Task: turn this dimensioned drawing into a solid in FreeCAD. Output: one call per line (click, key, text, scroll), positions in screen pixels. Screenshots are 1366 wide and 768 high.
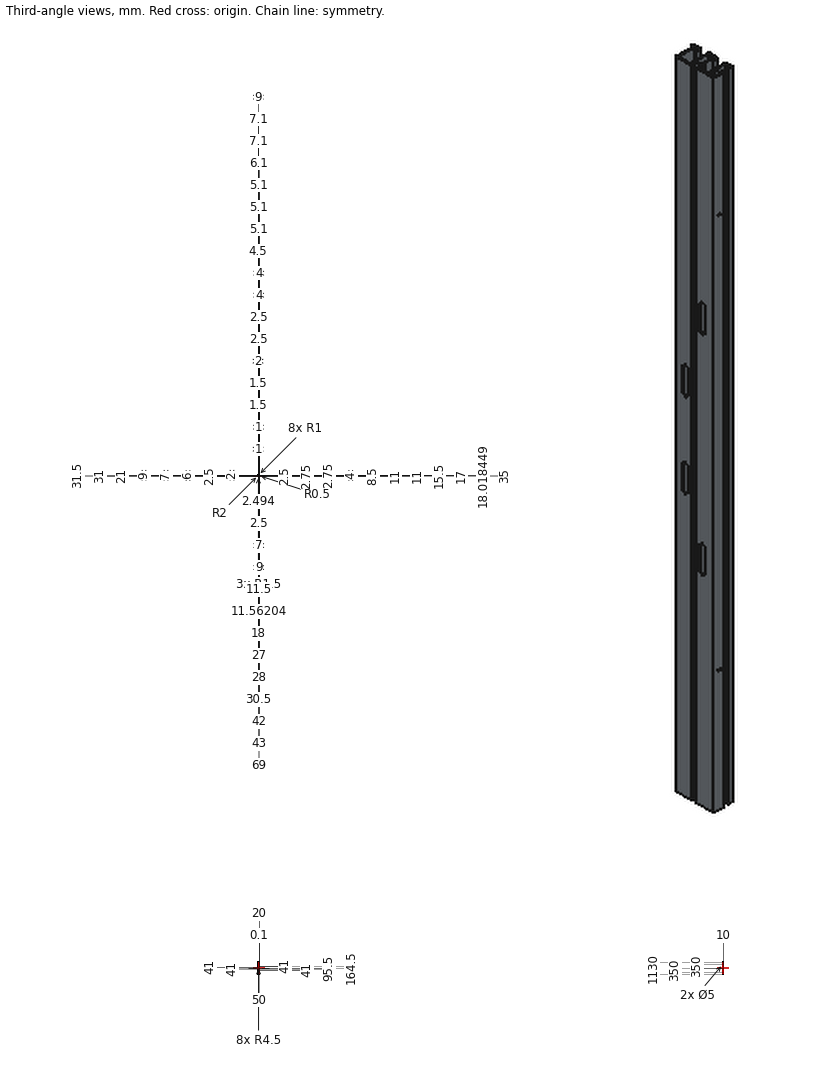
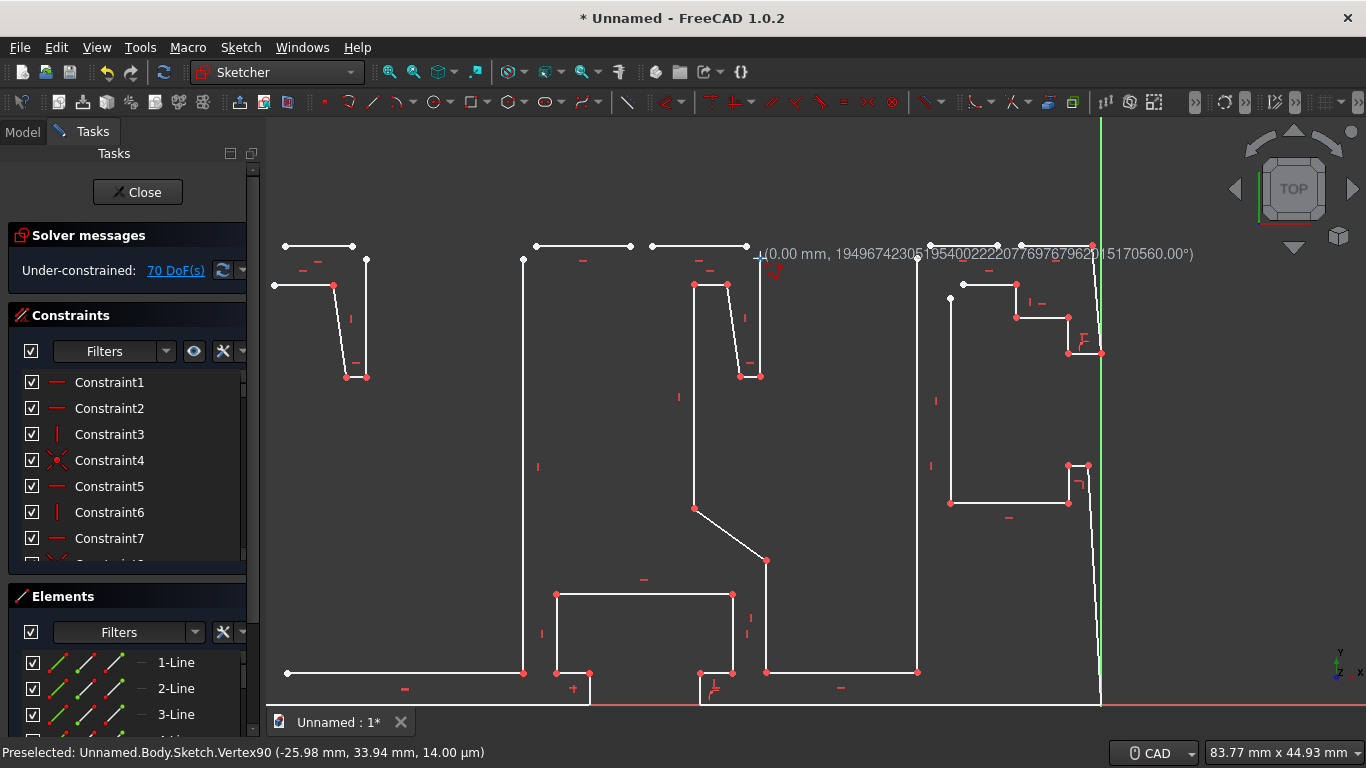
key(g)
key(3)
key(a)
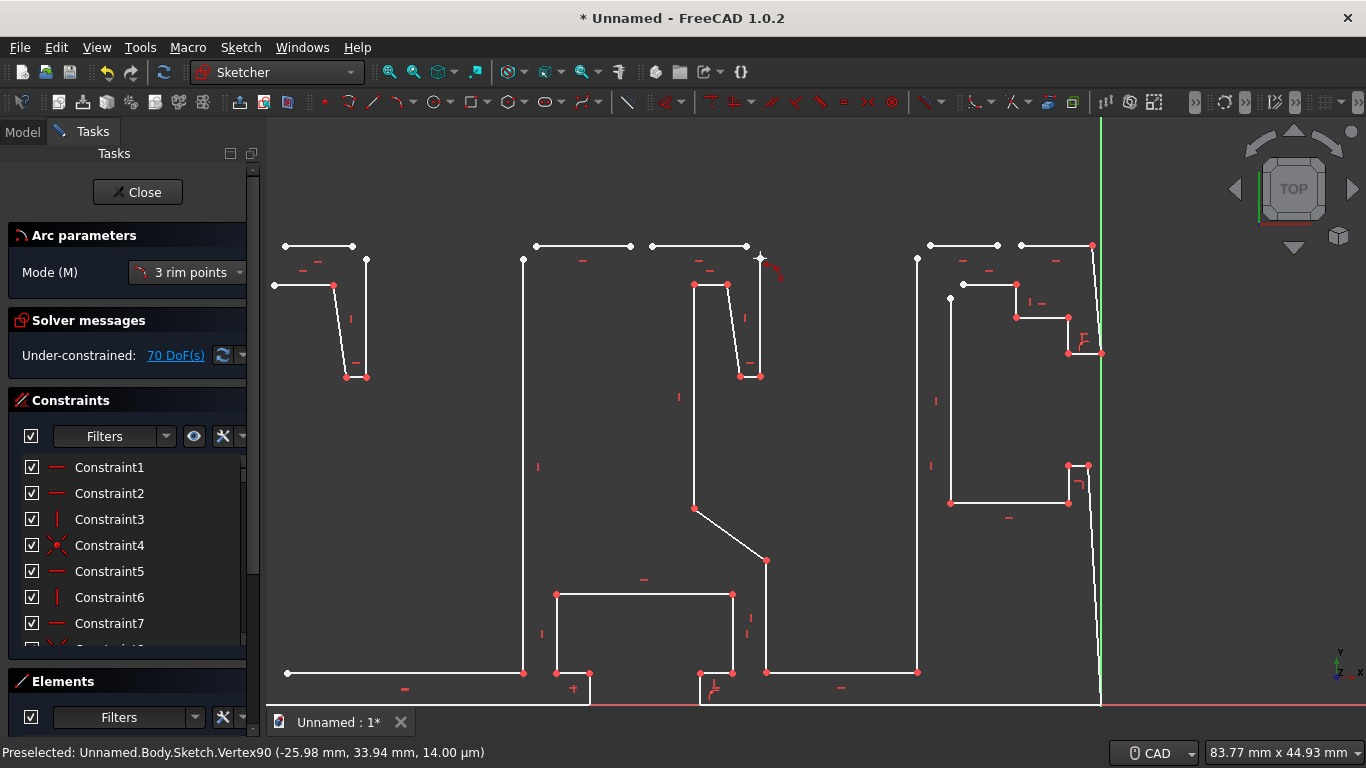
click(653, 246)
click(631, 246)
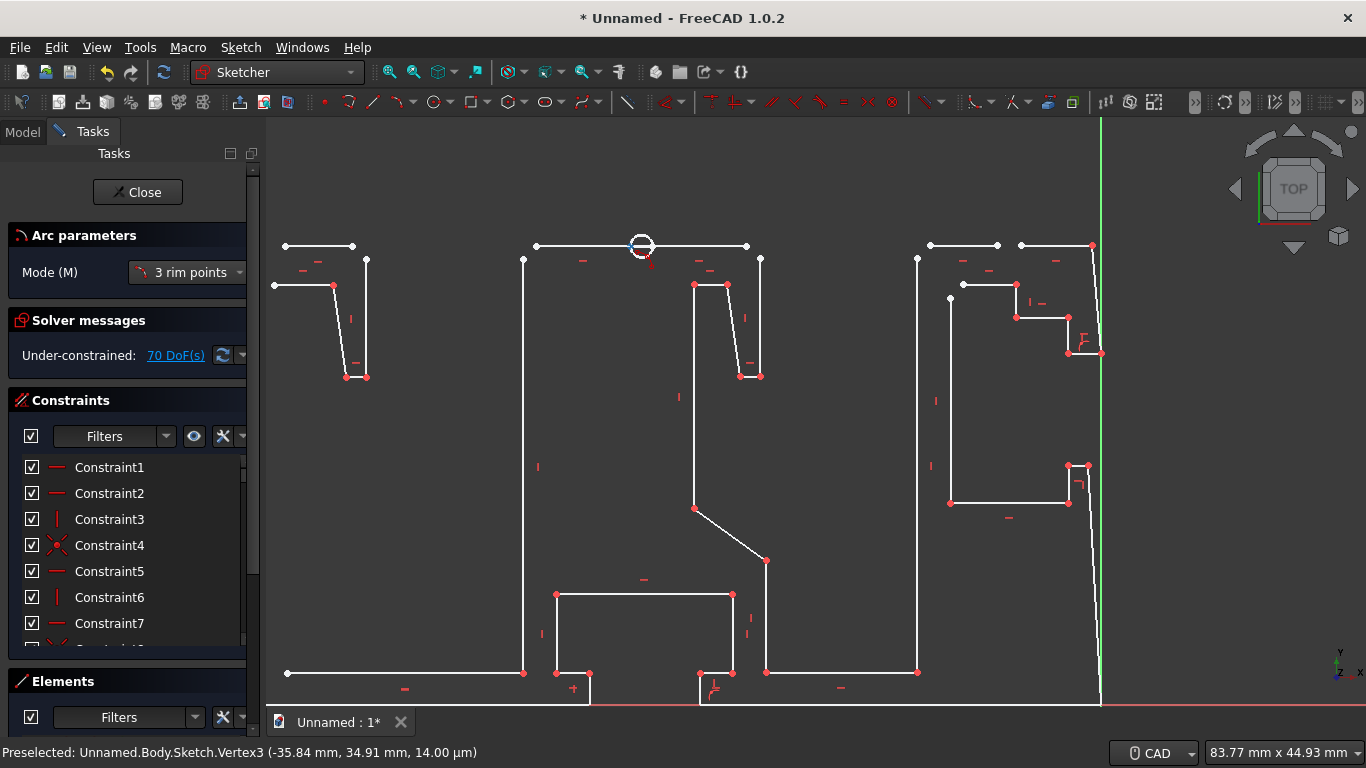
scroll(642, 249, up, 7)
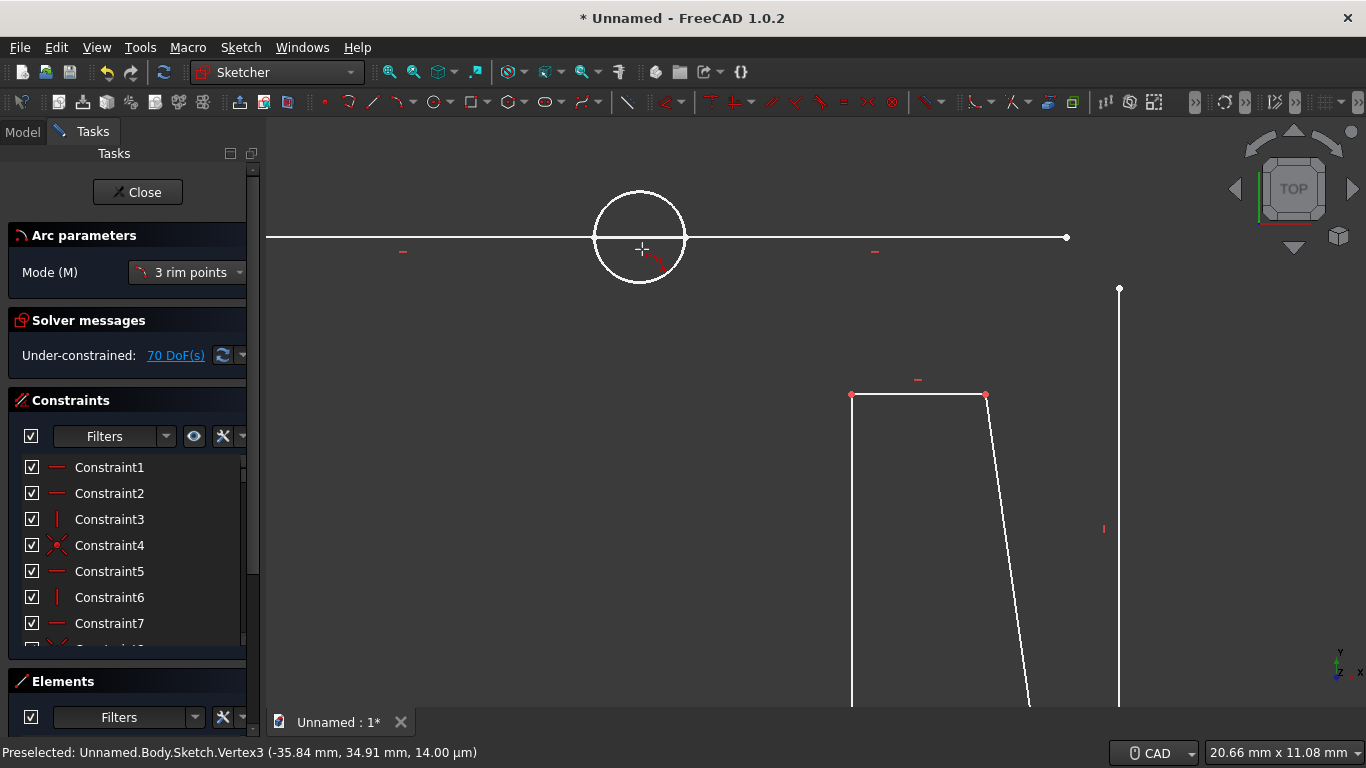
click(639, 248)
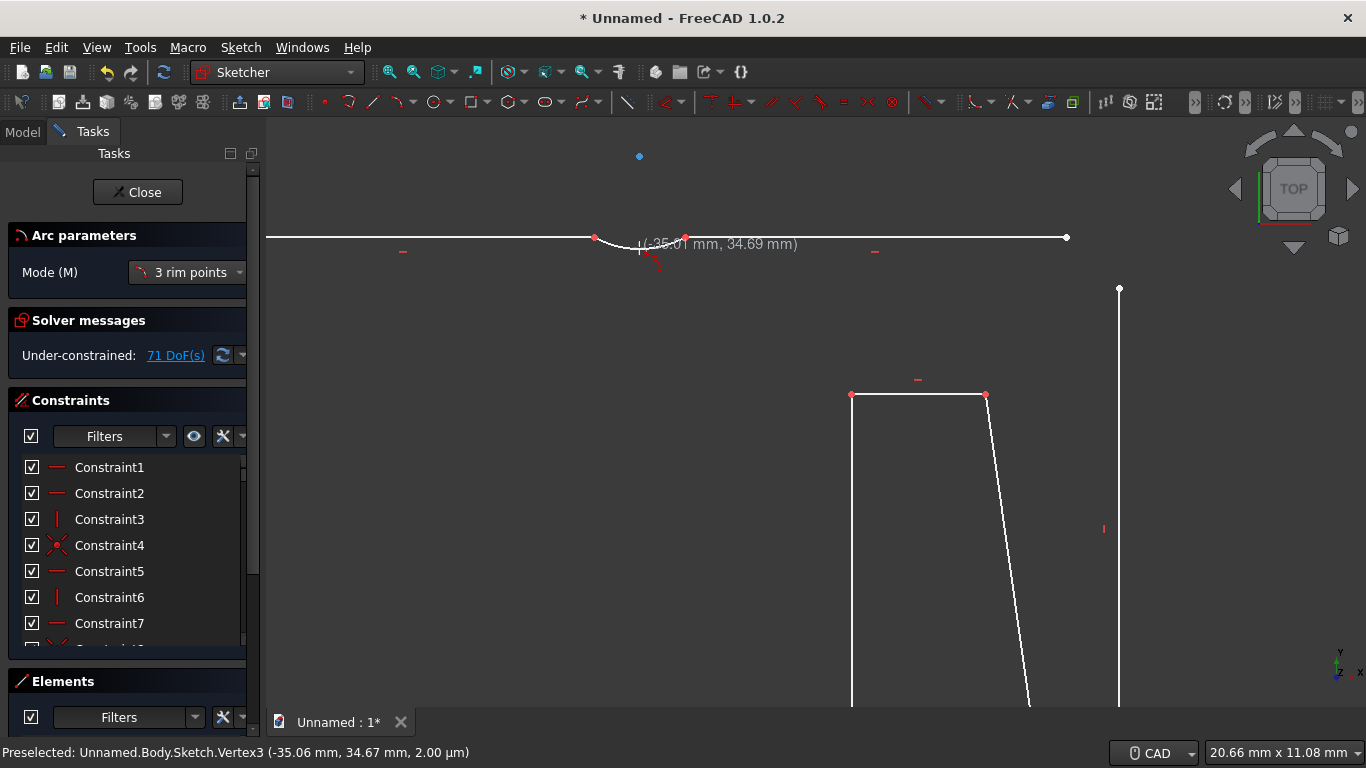
scroll(769, 263, down, 9)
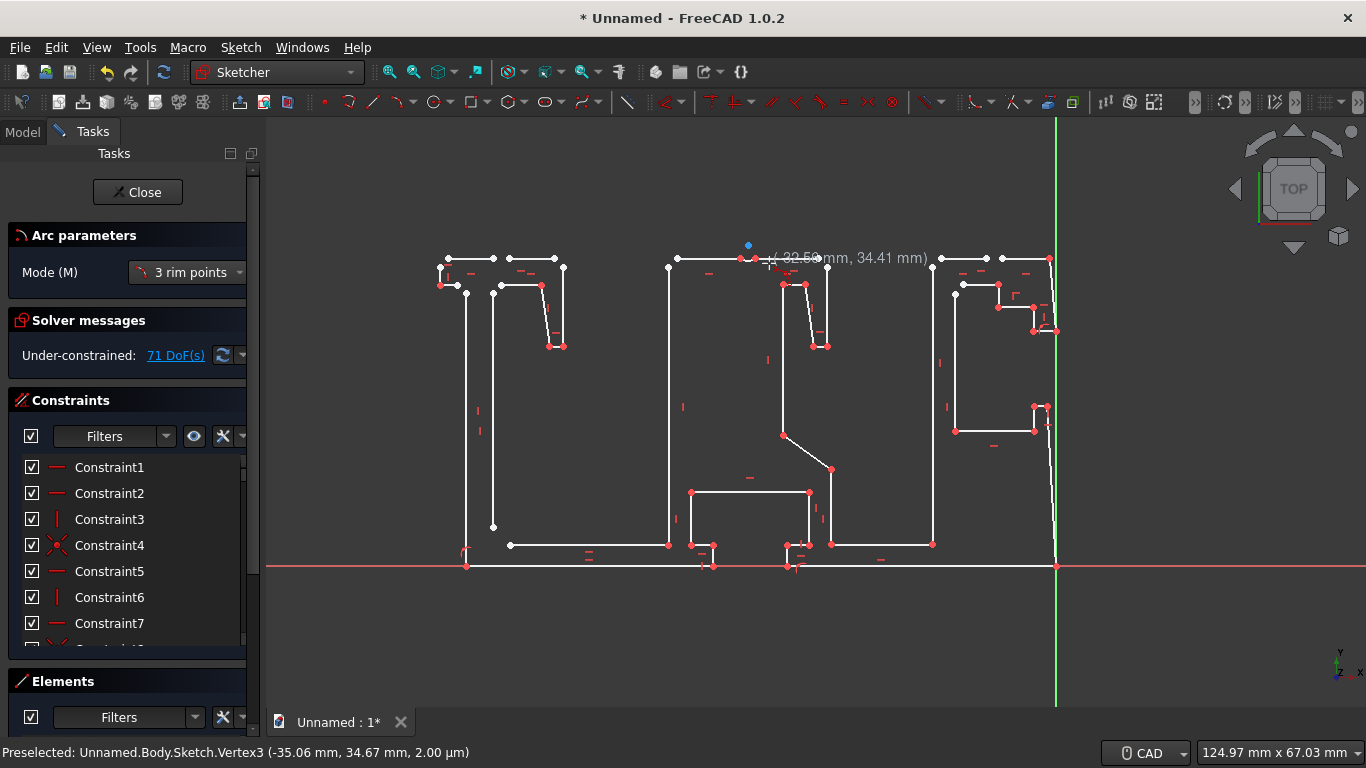
scroll(678, 258, up, 2)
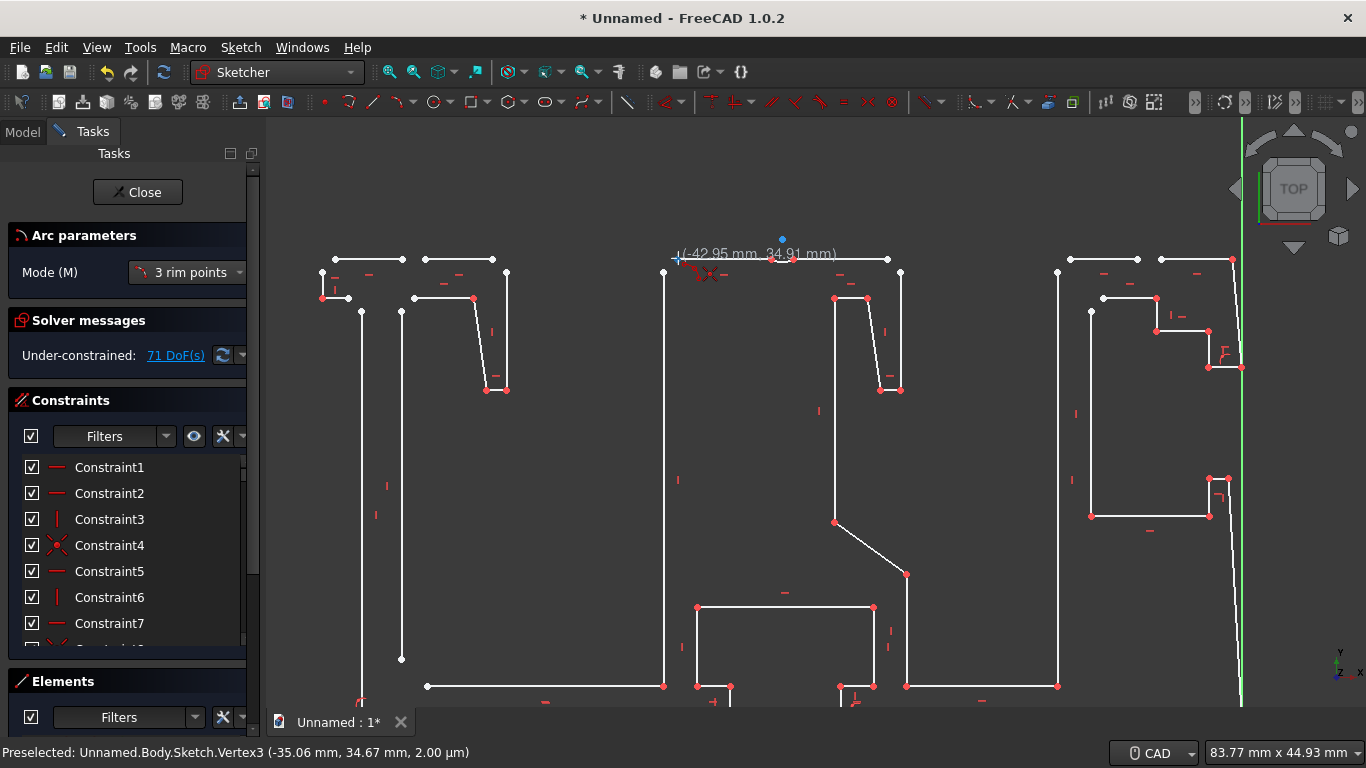
click(677, 259)
click(664, 272)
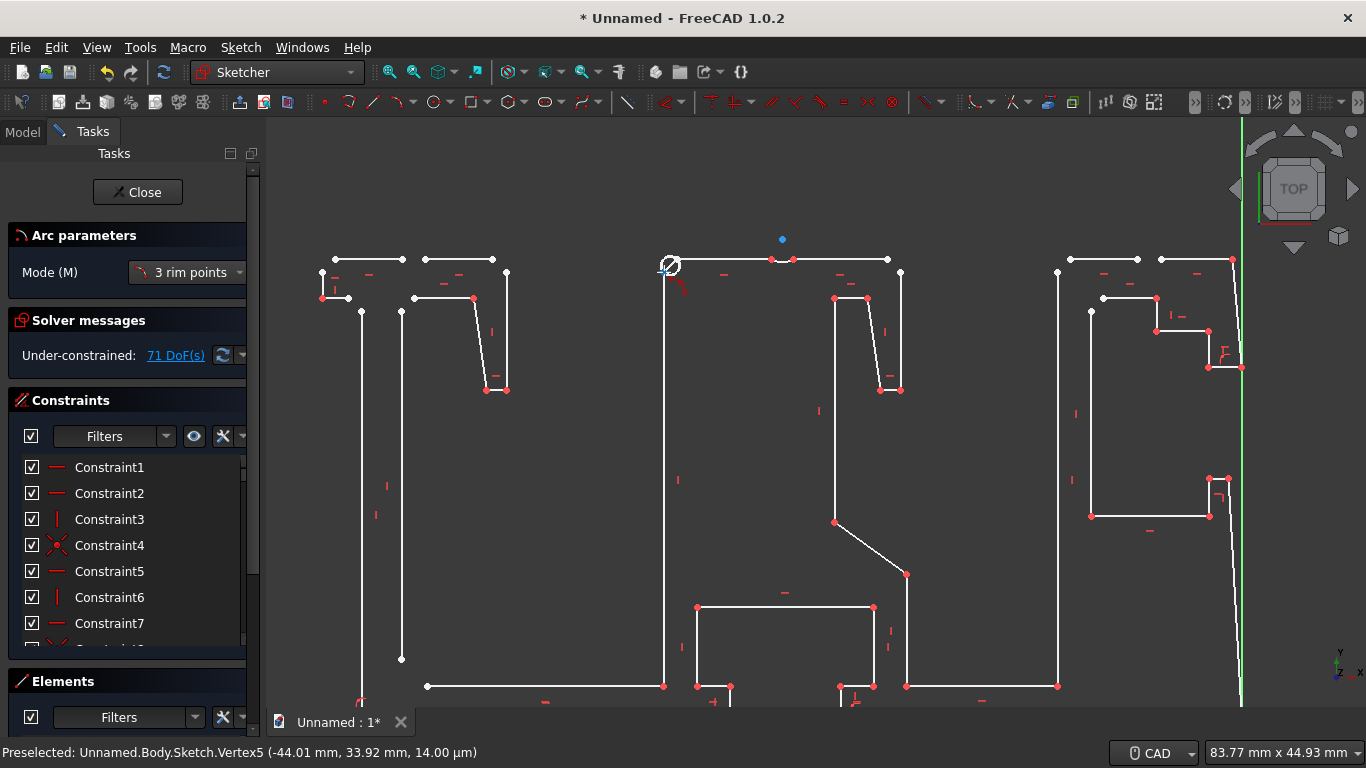
scroll(668, 262, up, 8)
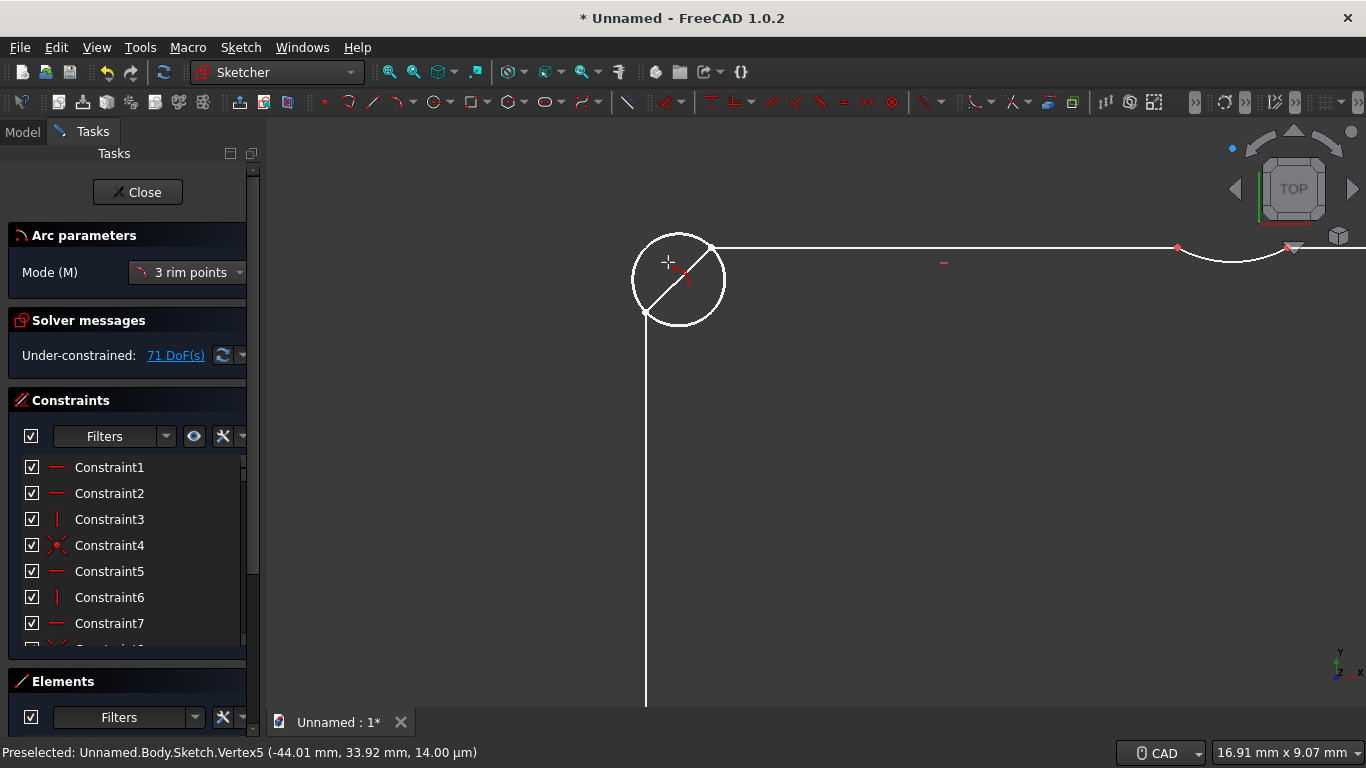
click(666, 261)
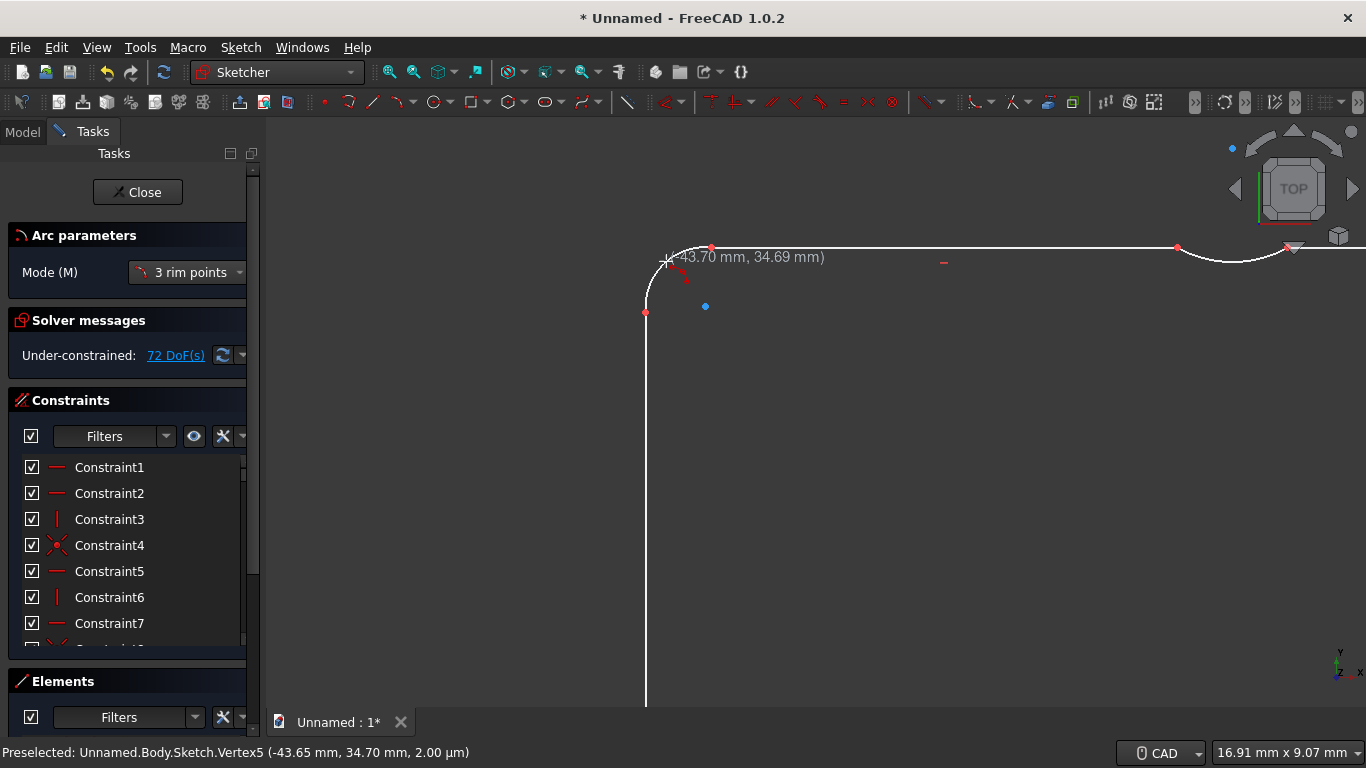
scroll(672, 260, down, 10)